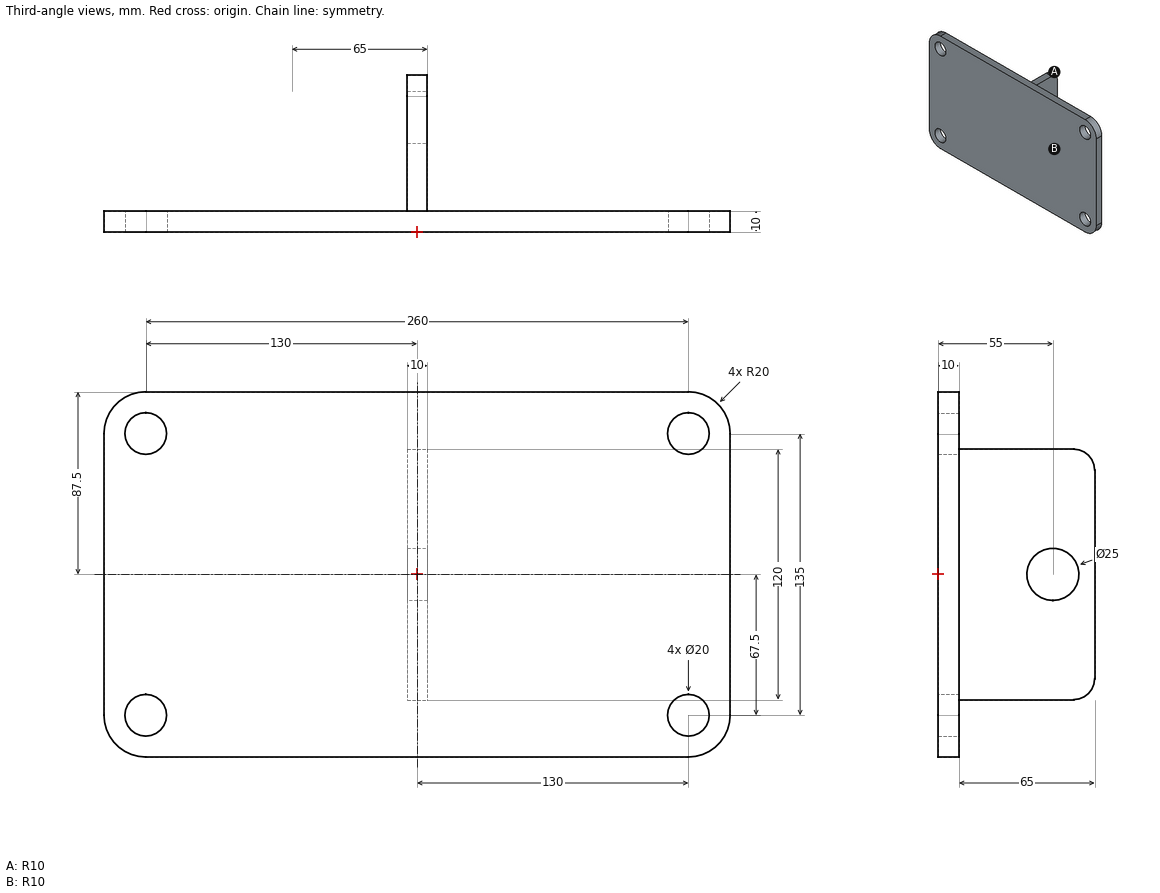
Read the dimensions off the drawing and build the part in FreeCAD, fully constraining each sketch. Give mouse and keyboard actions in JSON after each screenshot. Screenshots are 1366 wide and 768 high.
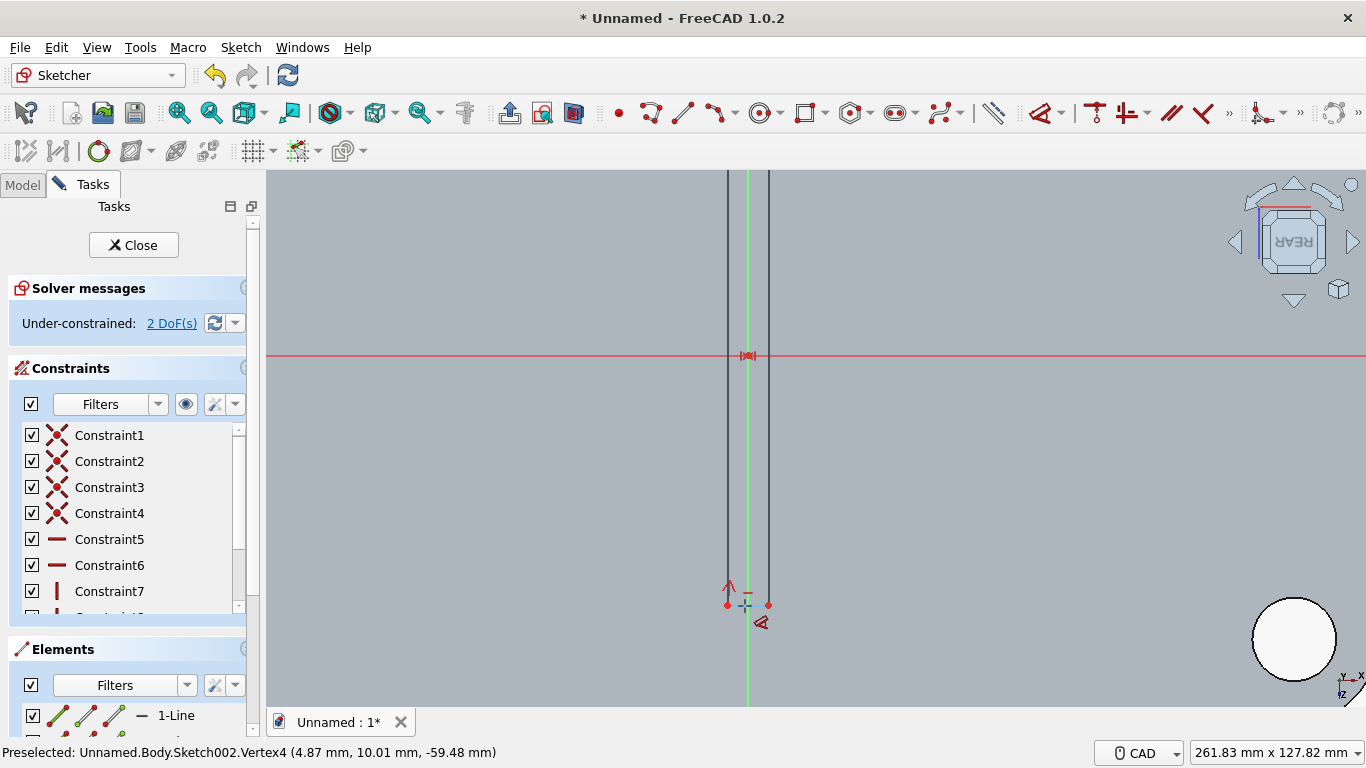
{"action": "left_click", "coordinate": [744, 606]}
{"action": "left_click", "coordinate": [734, 640]}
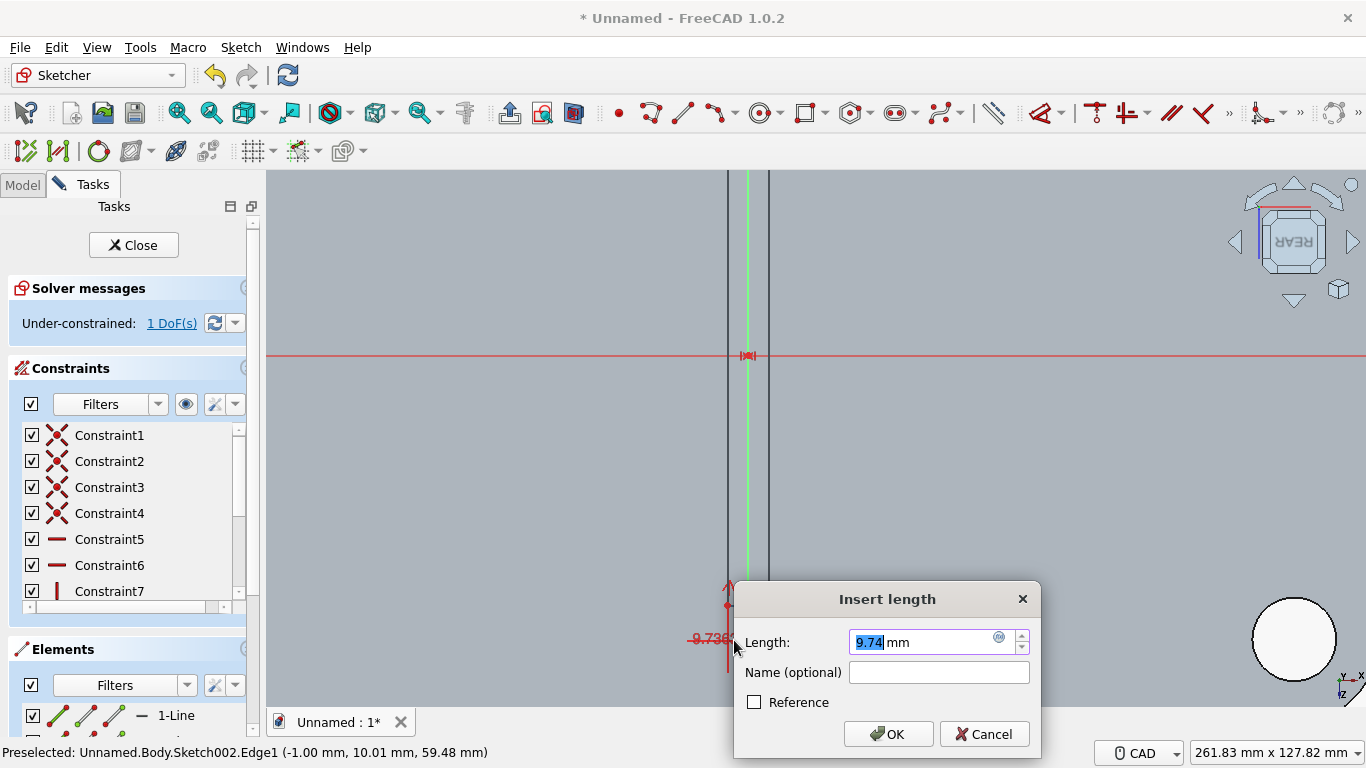
{"action": "type", "text": "10"}
{"action": "key", "text": "Return"}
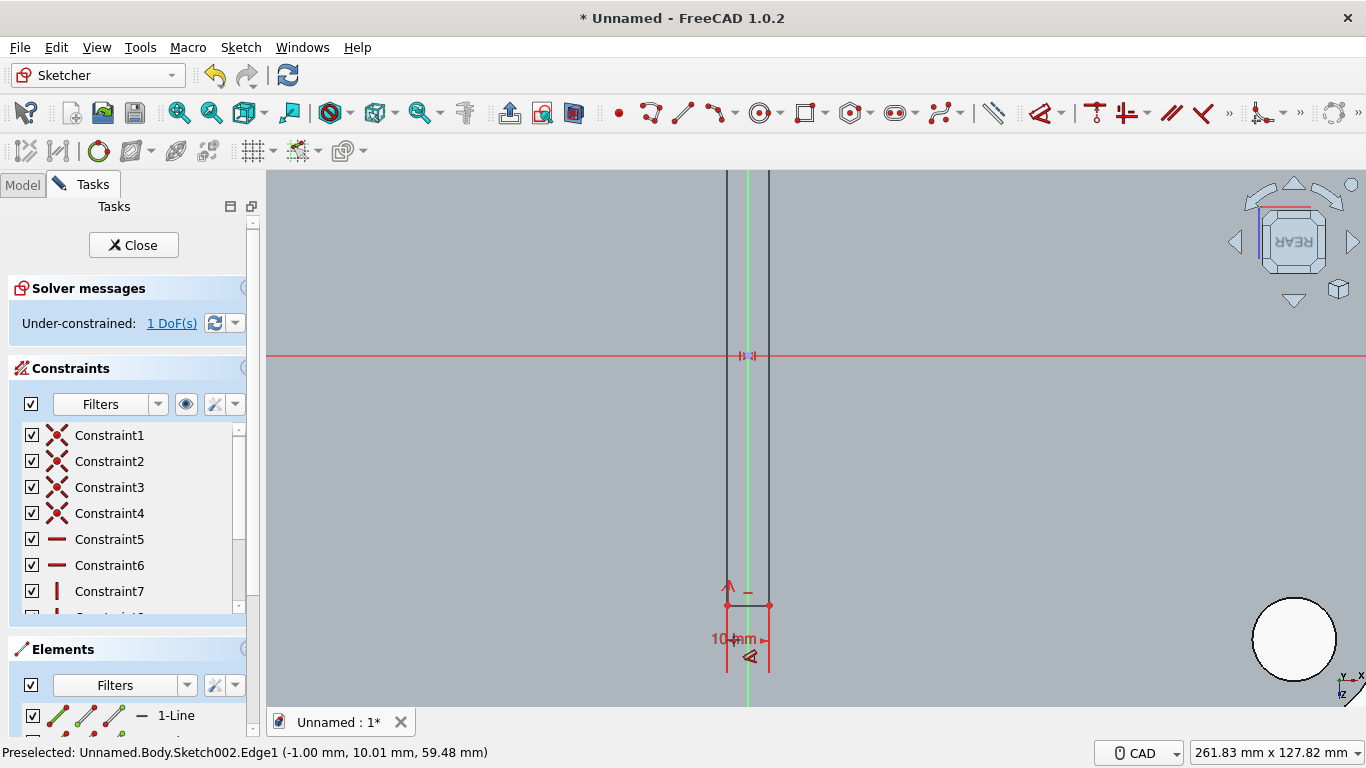
{"action": "left_click", "coordinate": [769, 456]}
{"action": "left_click", "coordinate": [803, 402]}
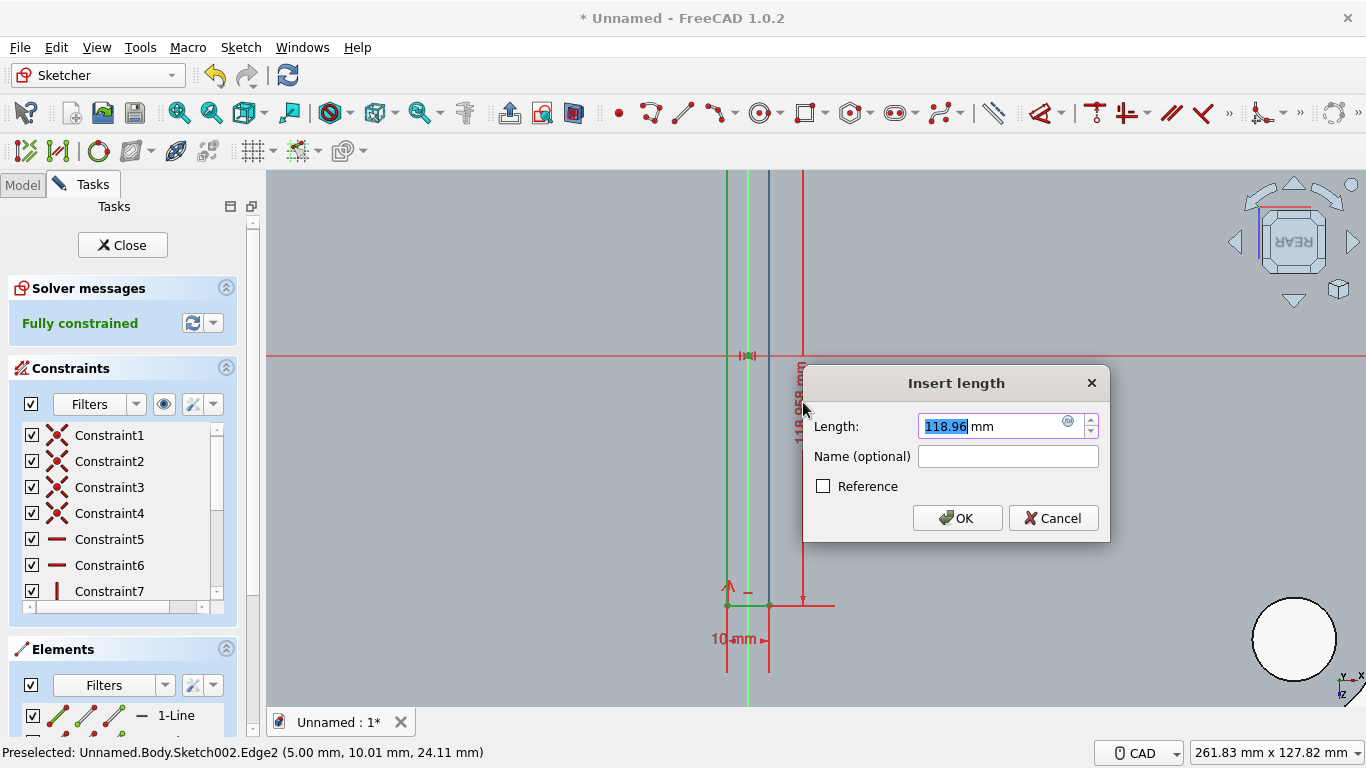
{"action": "type", "text": "120"}
{"action": "key", "text": "Return"}
{"action": "key", "text": "Escape"}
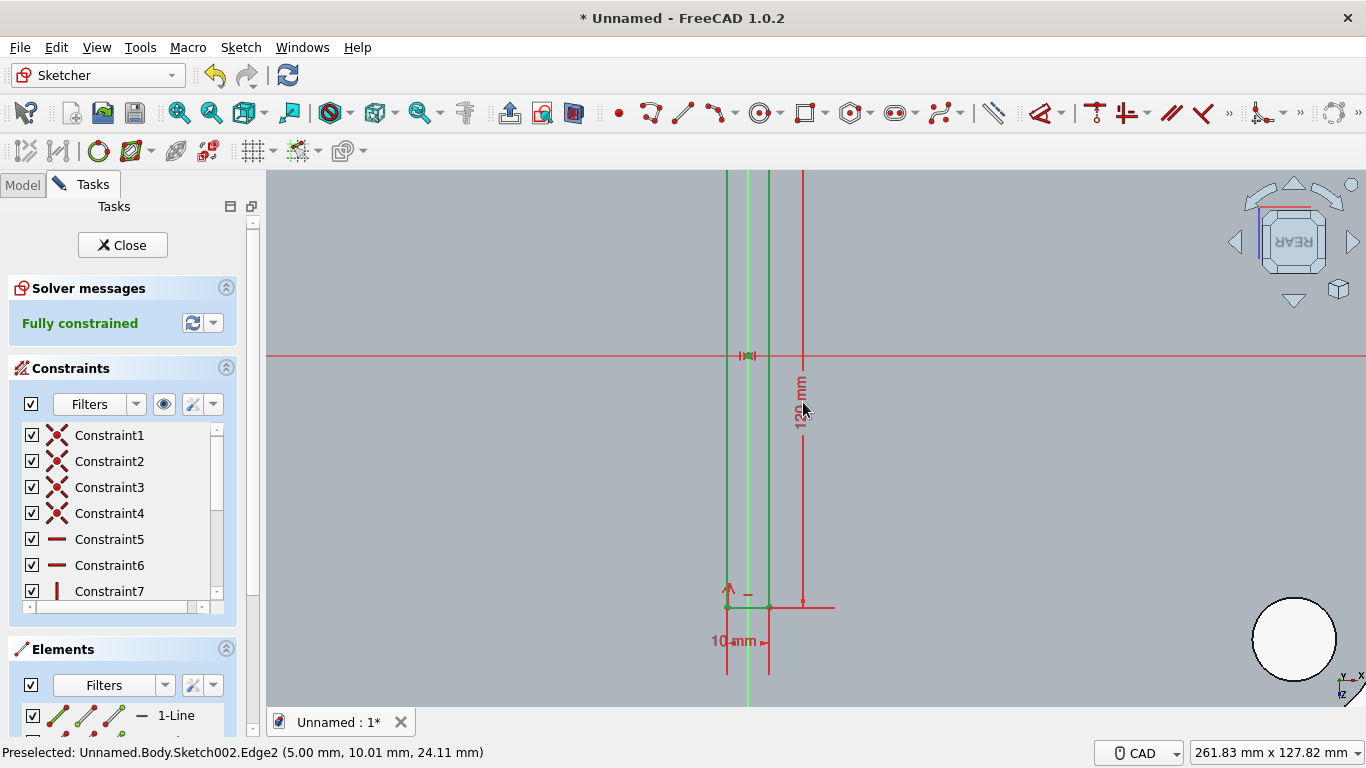
{"action": "left_click", "coordinate": [123, 245]}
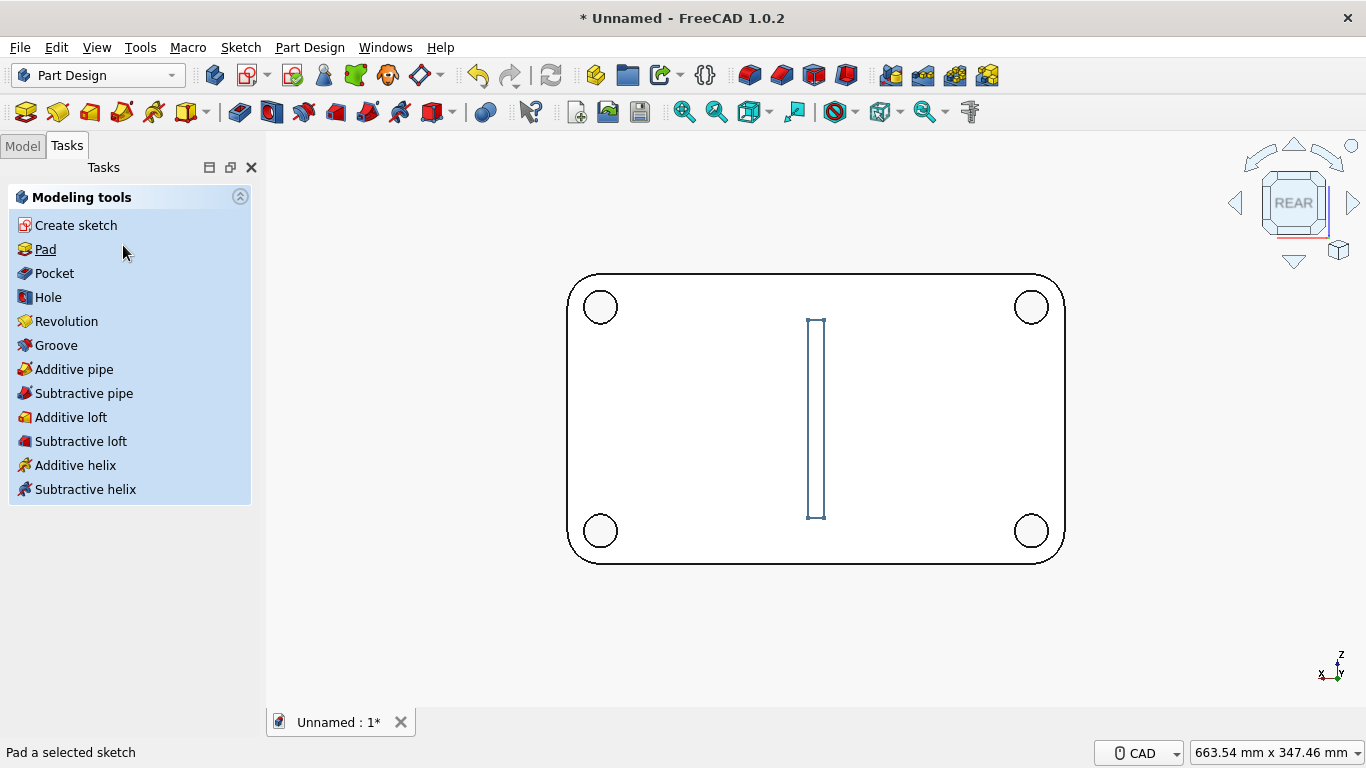
{"action": "left_click", "coordinate": [26, 112]}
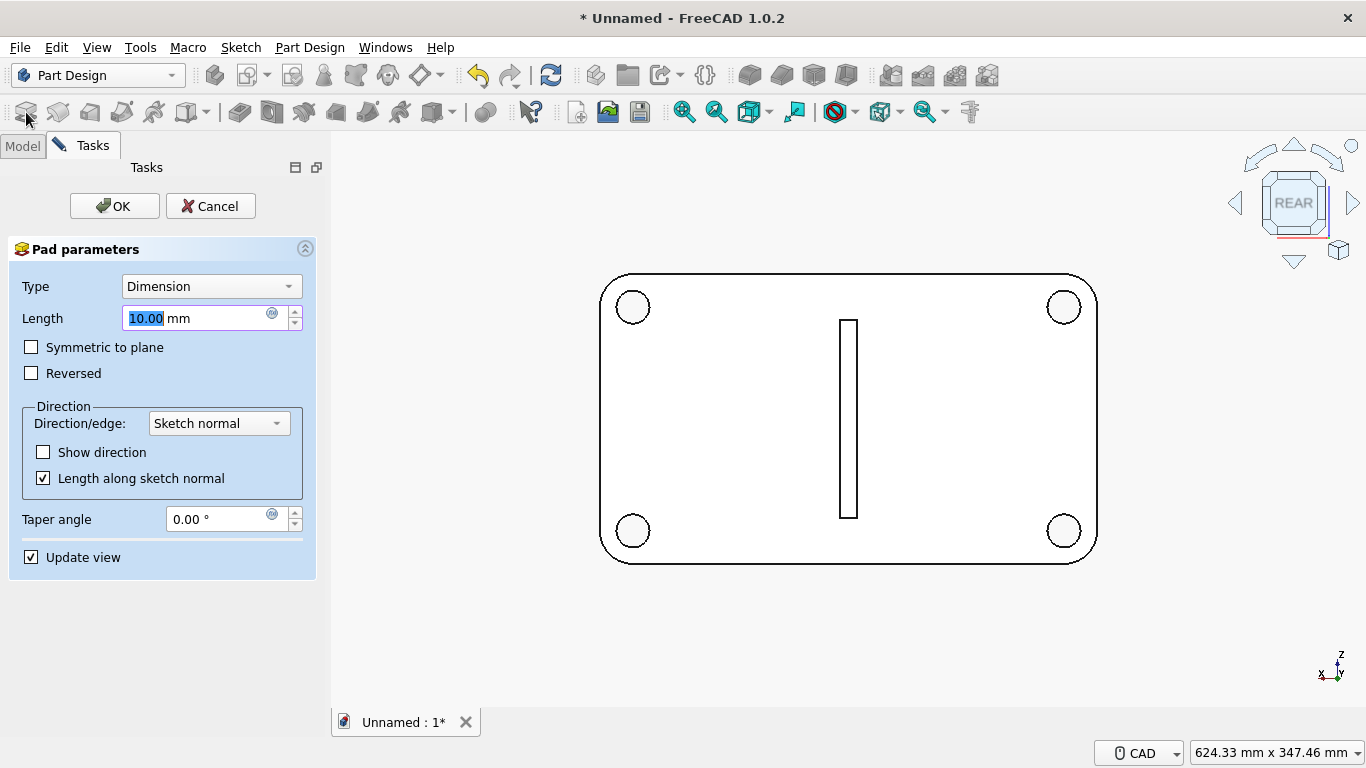
{"action": "type", "text": "65"}
{"action": "key", "text": "Tab"}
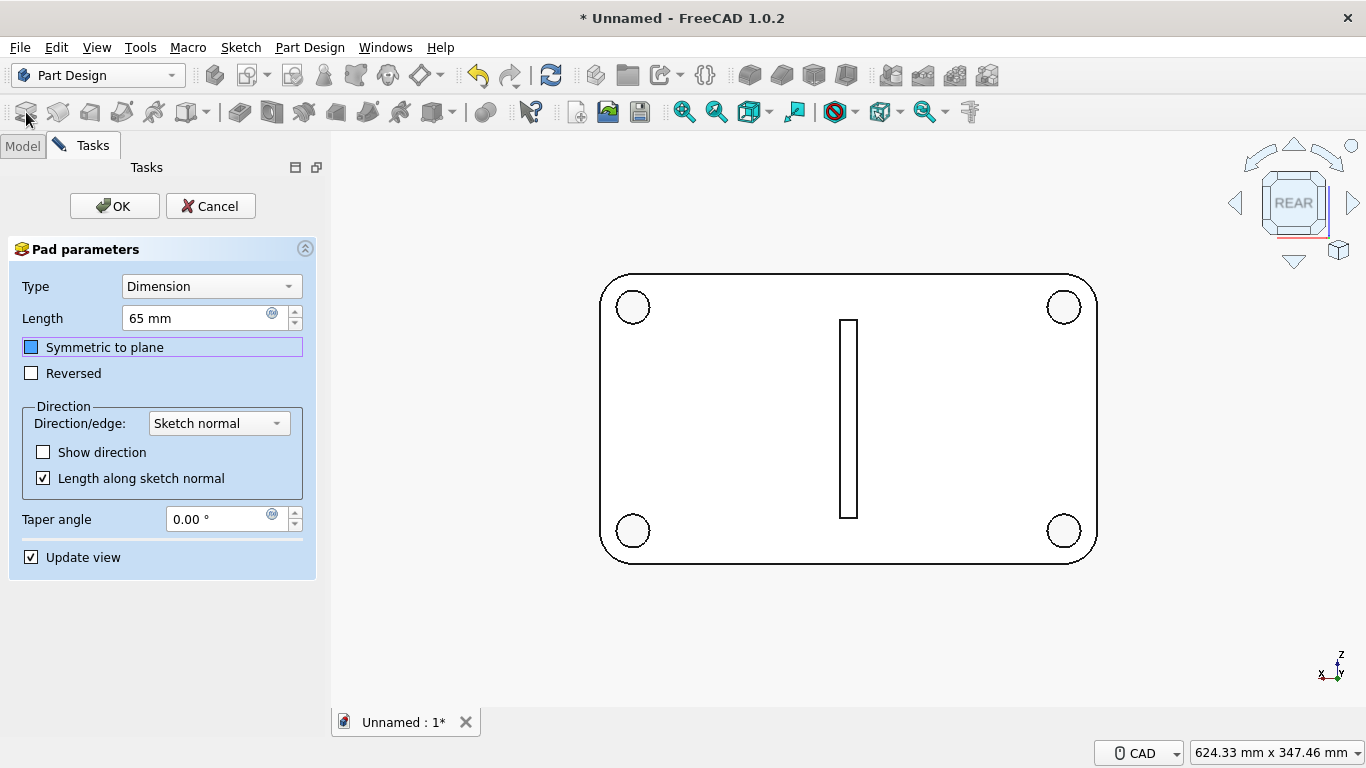
{"action": "left_click", "coordinate": [115, 206]}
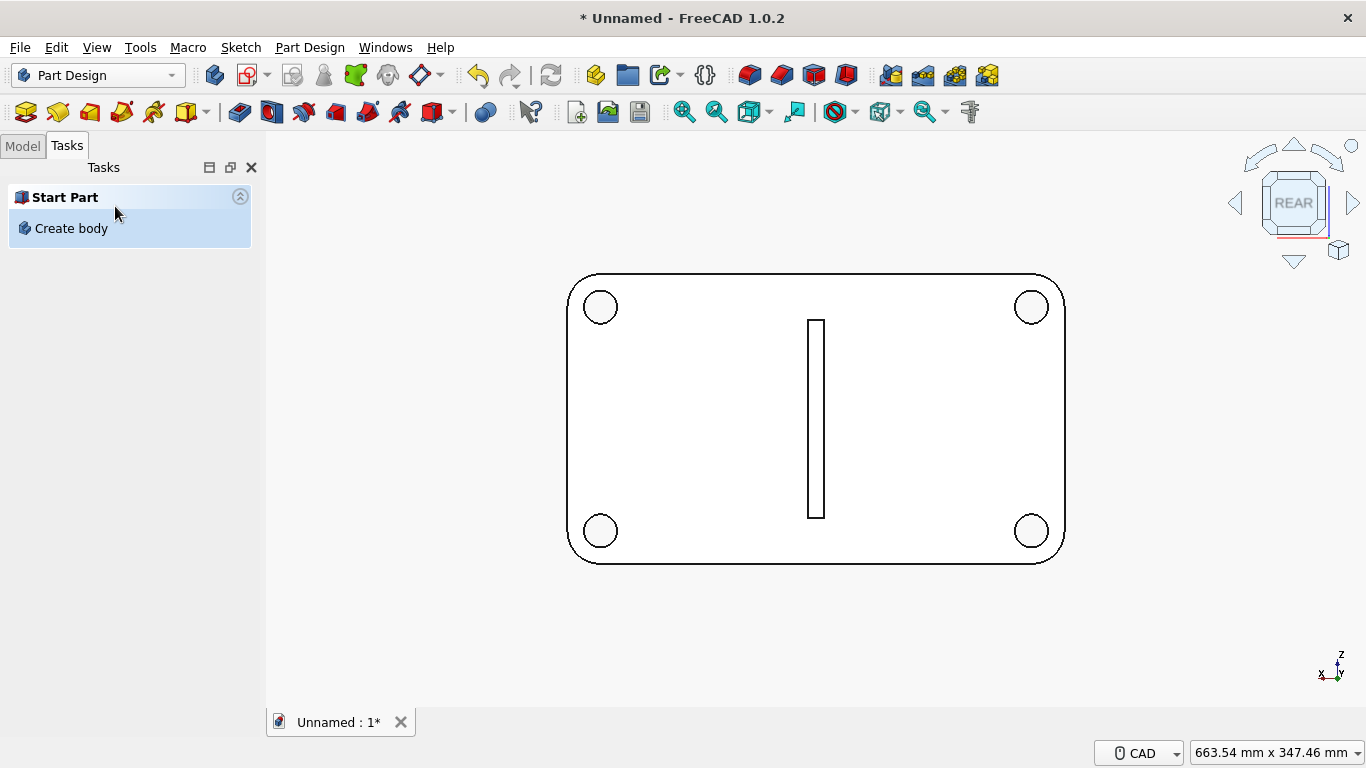
{"action": "scroll", "coordinate": [816, 319], "scroll_direction": "up", "scroll_amount": 5}